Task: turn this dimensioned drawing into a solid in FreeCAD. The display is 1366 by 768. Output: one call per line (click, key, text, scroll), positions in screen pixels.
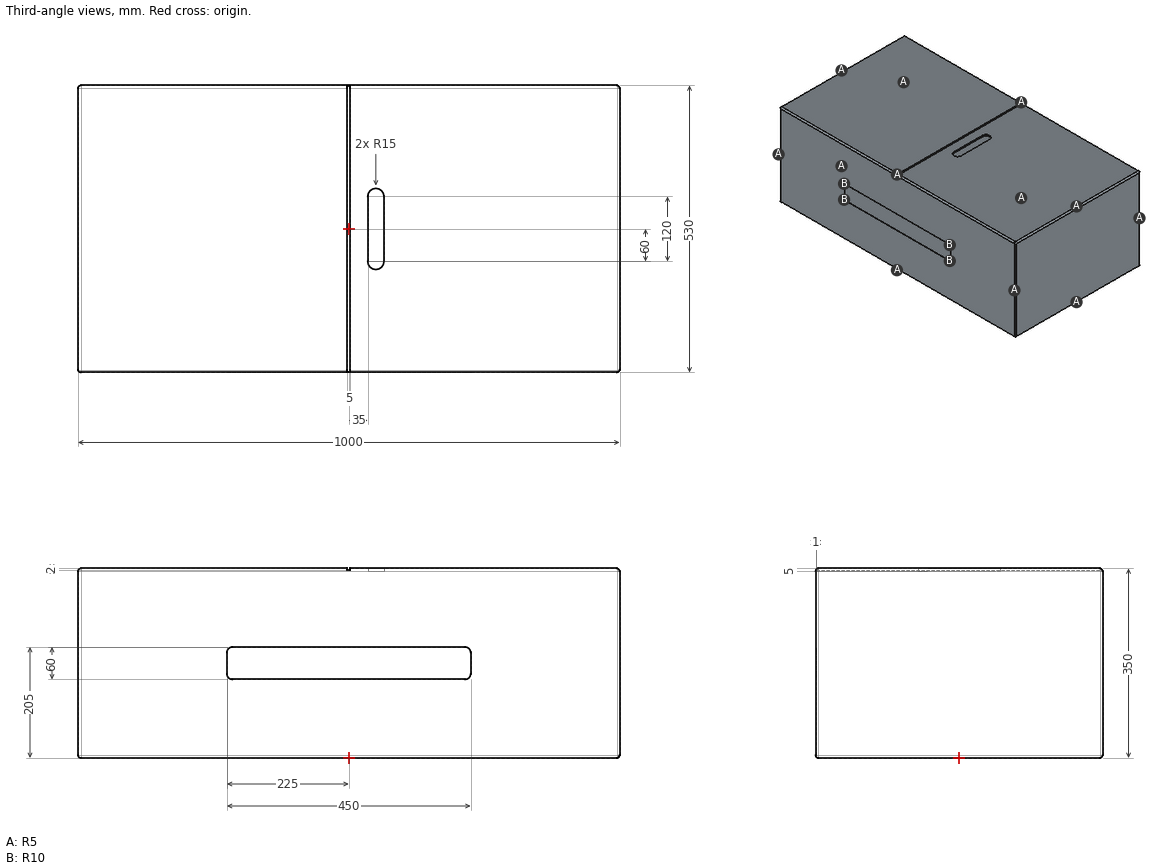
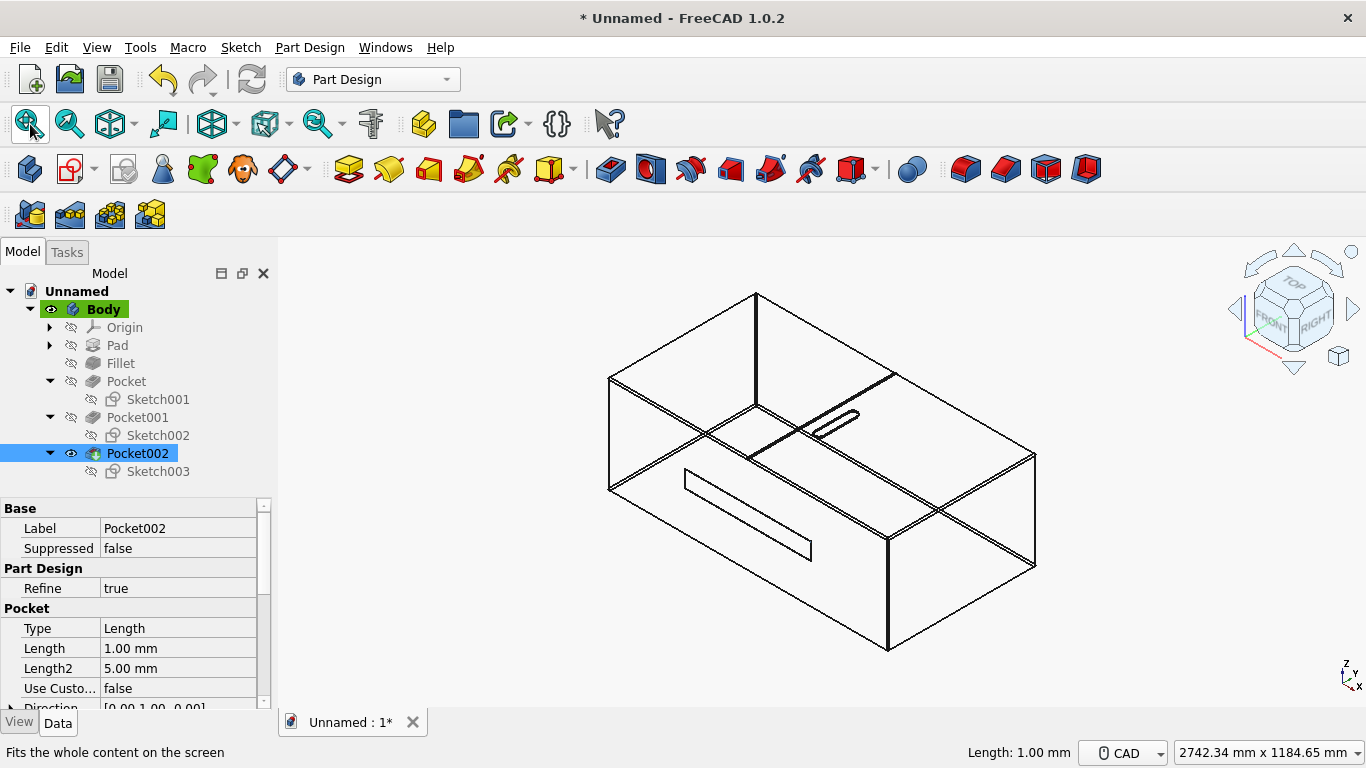
key(2)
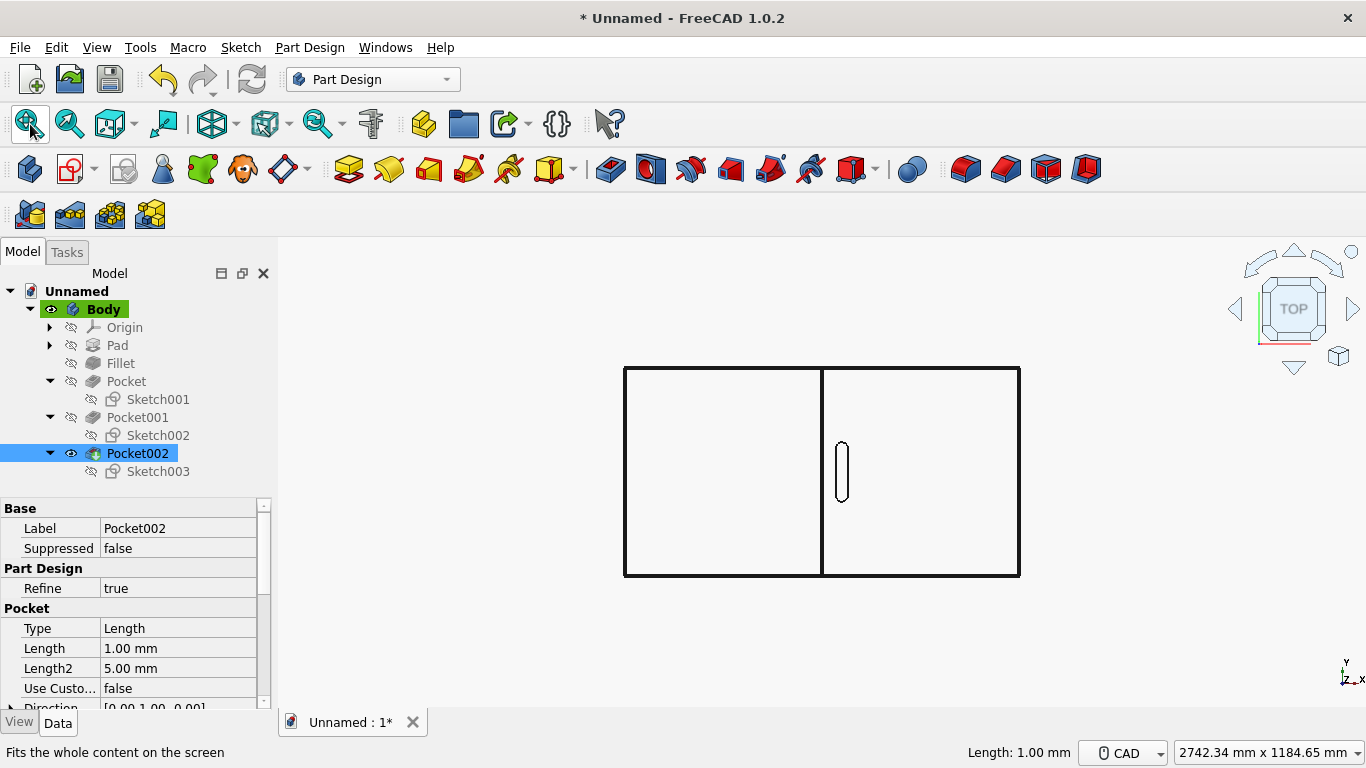
click(30, 124)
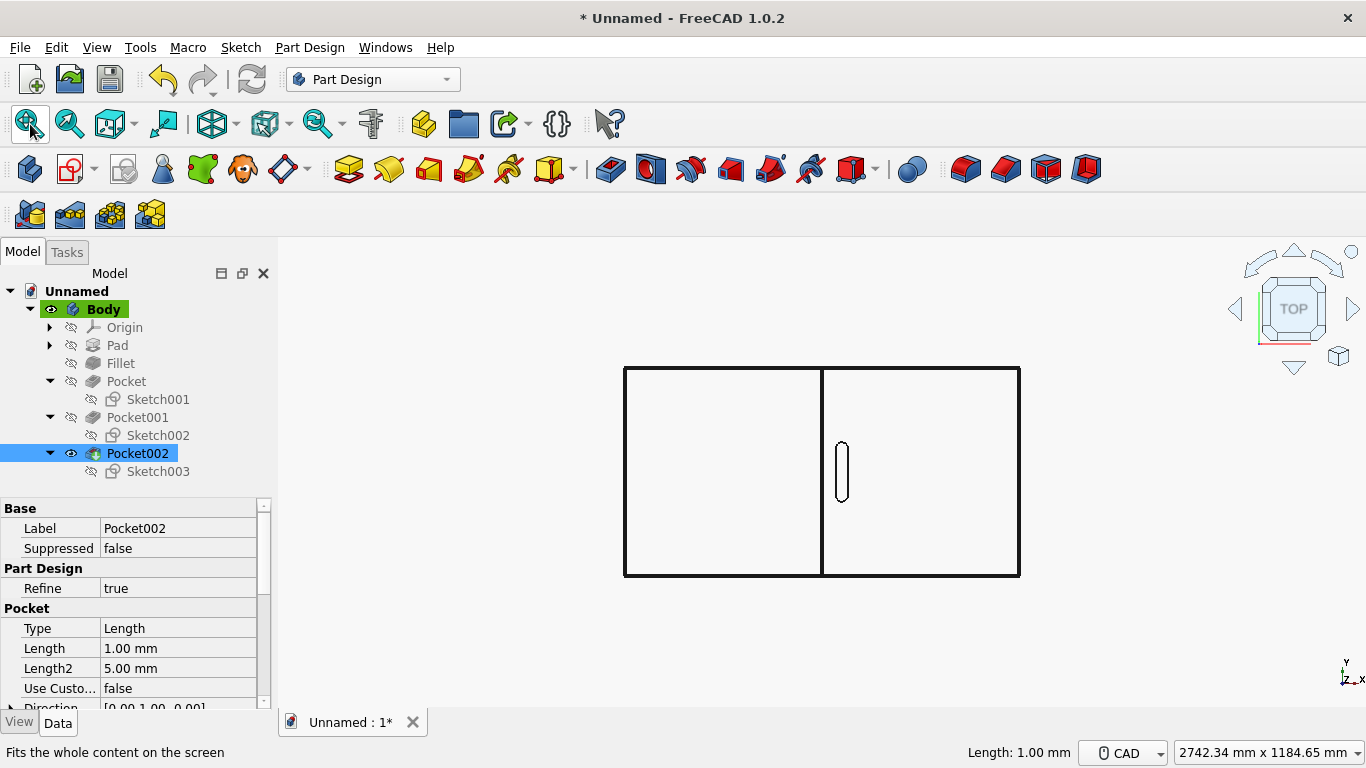
scroll(911, 576, up, 15)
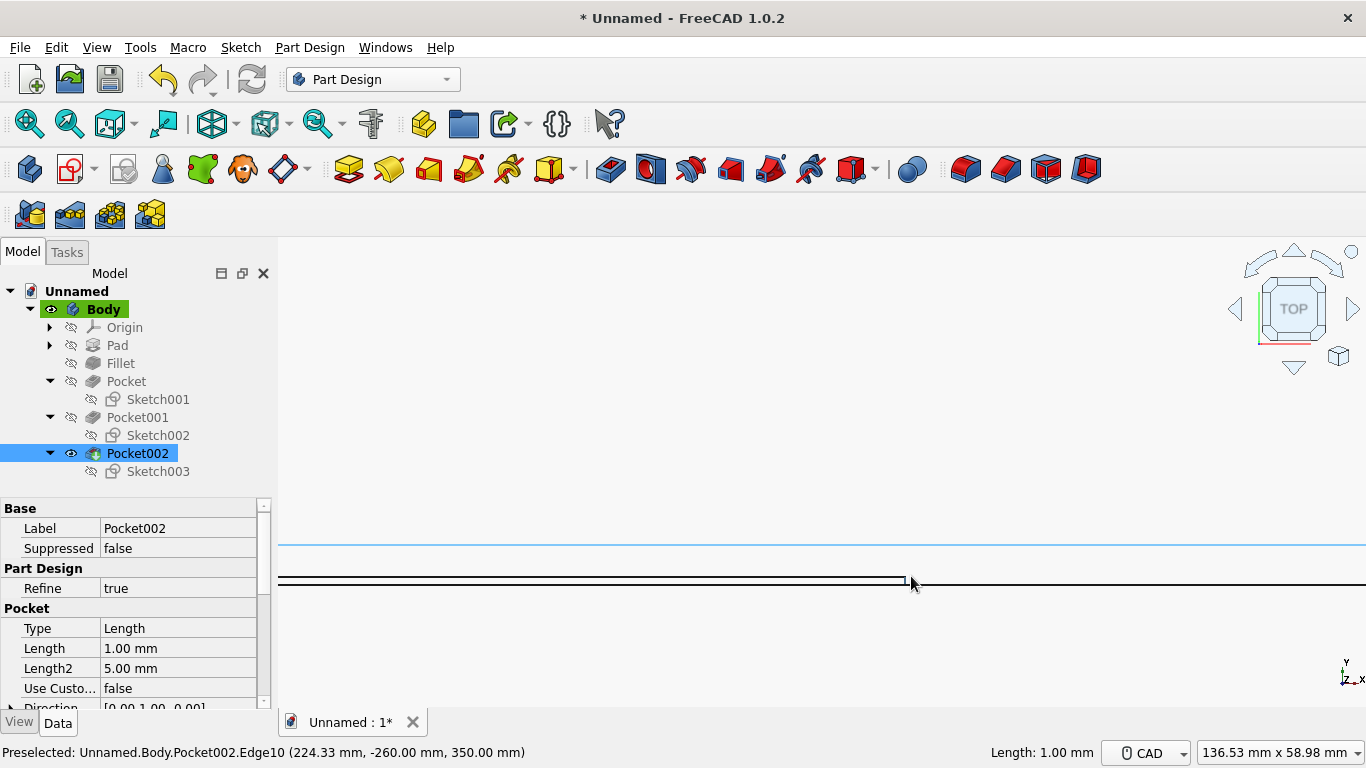
scroll(905, 580, up, 9)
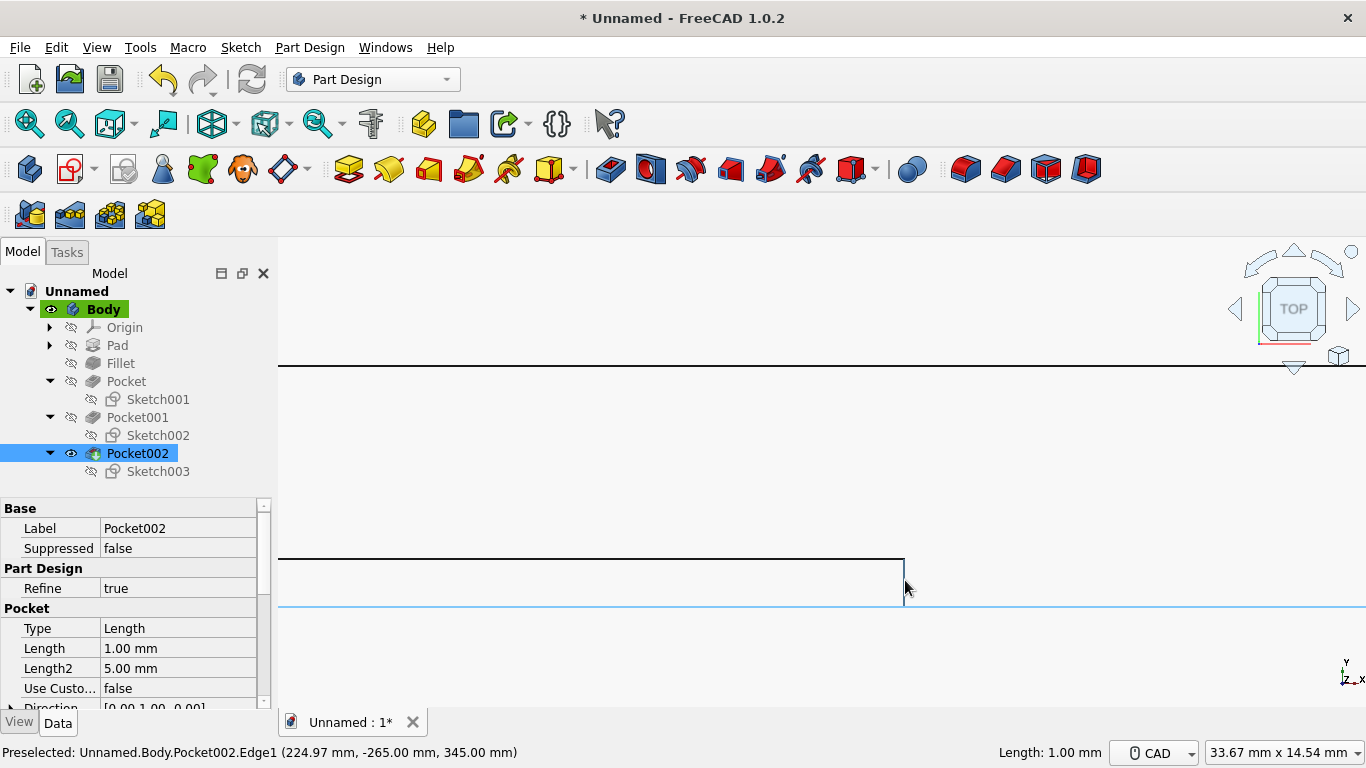
click(30, 124)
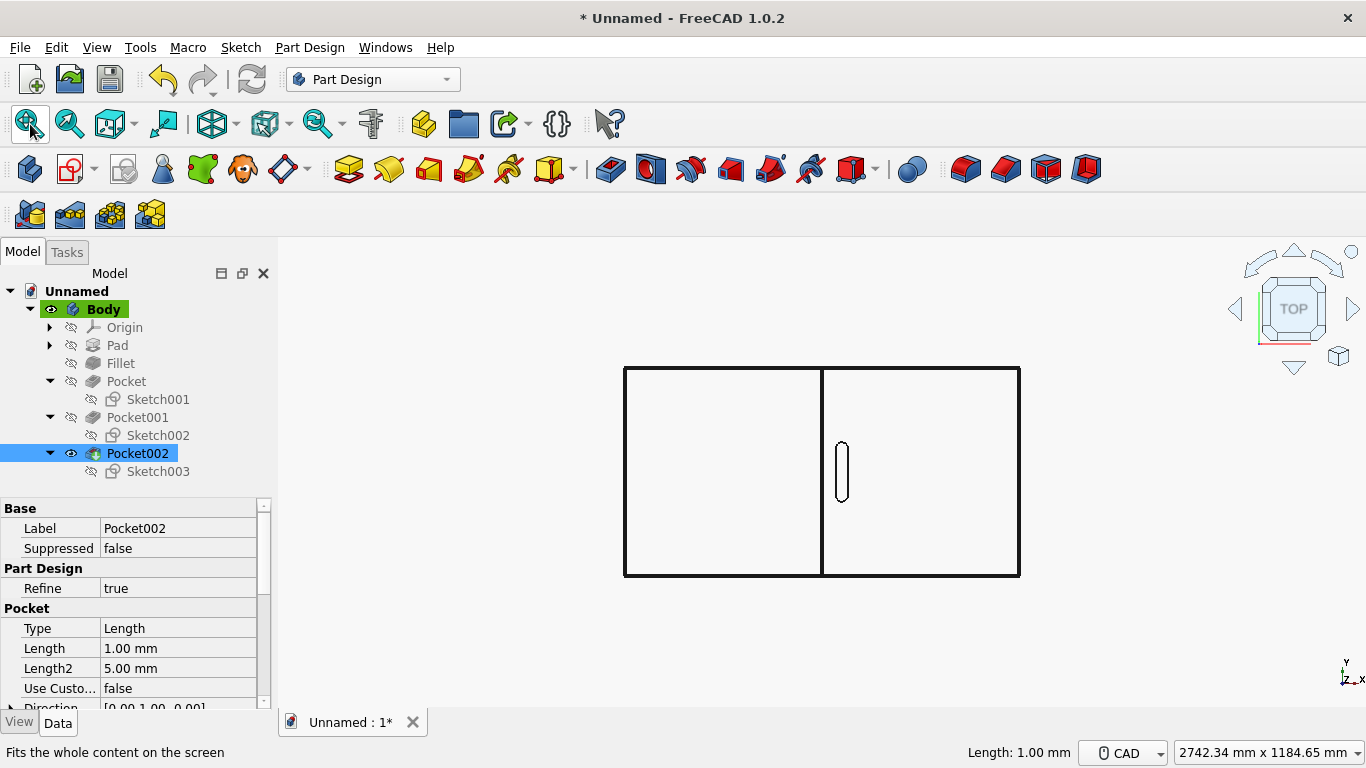
key(1)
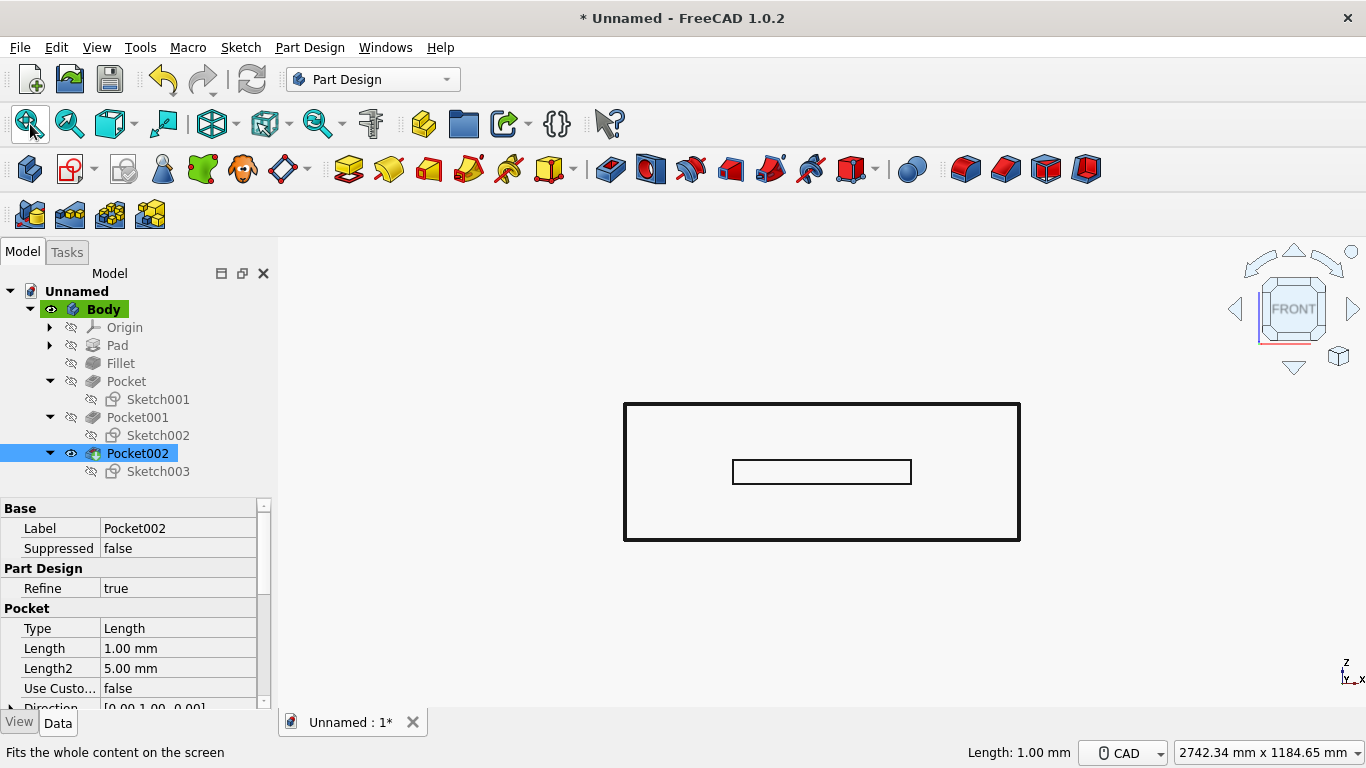
click(30, 124)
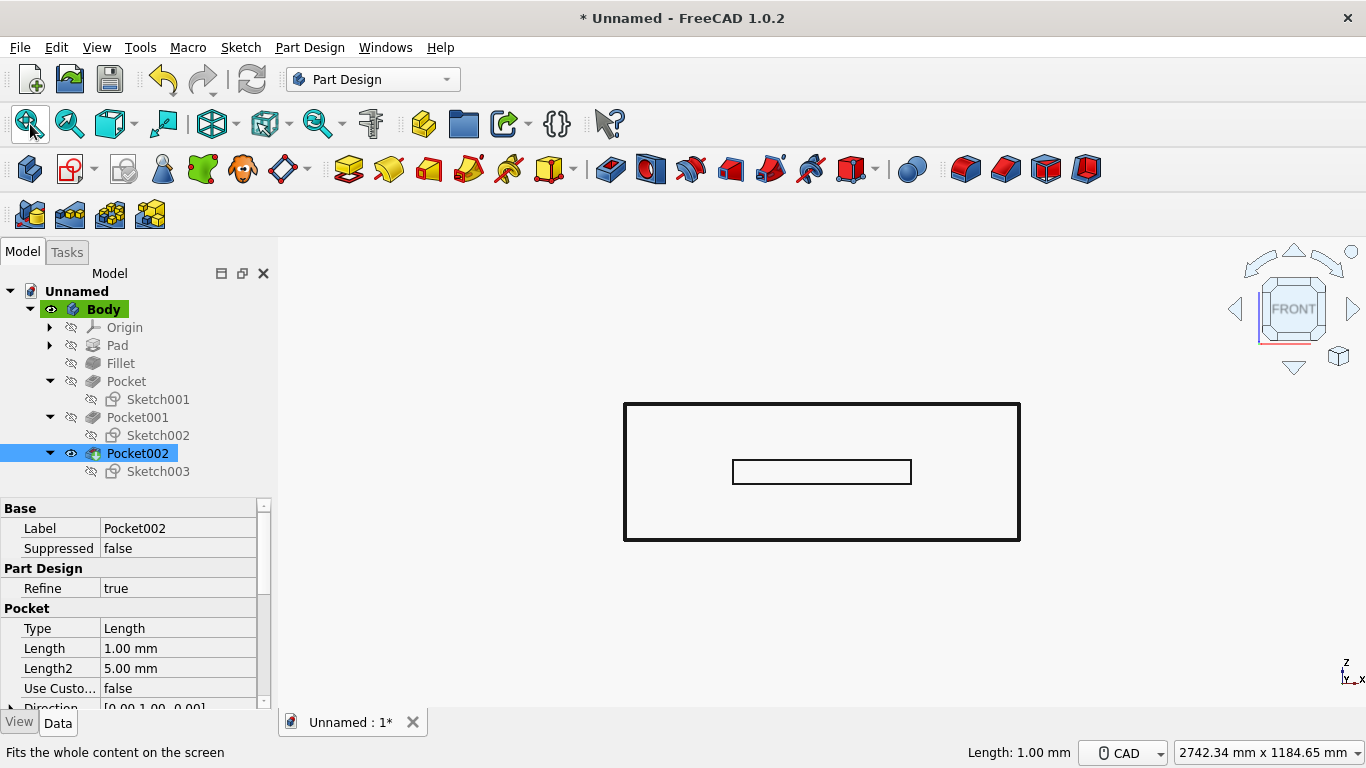
scroll(911, 483, up, 15)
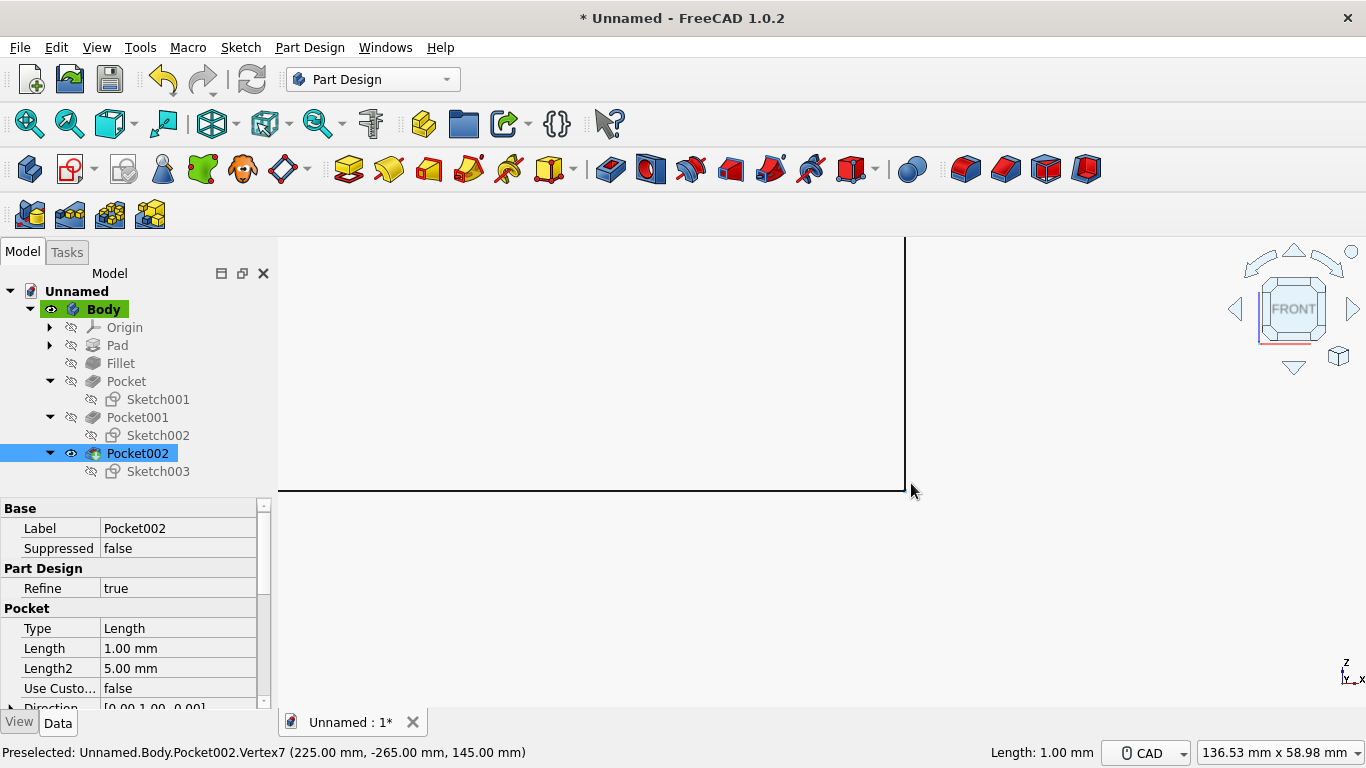
scroll(905, 490, up, 9)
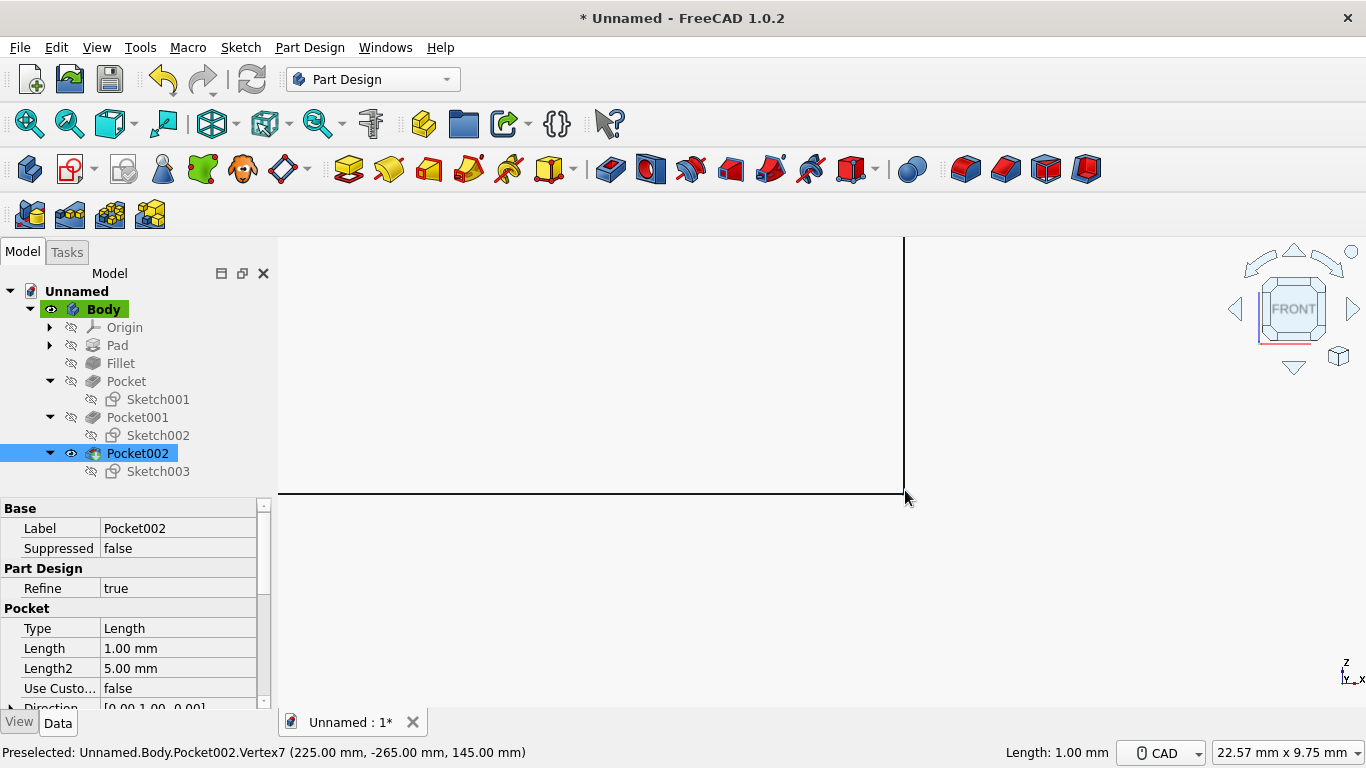
click(30, 124)